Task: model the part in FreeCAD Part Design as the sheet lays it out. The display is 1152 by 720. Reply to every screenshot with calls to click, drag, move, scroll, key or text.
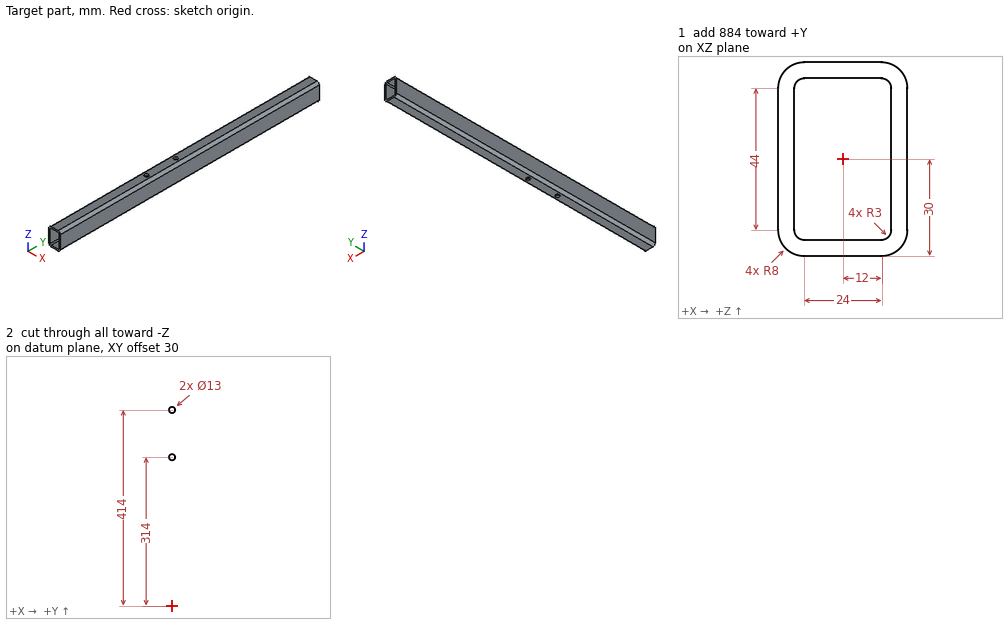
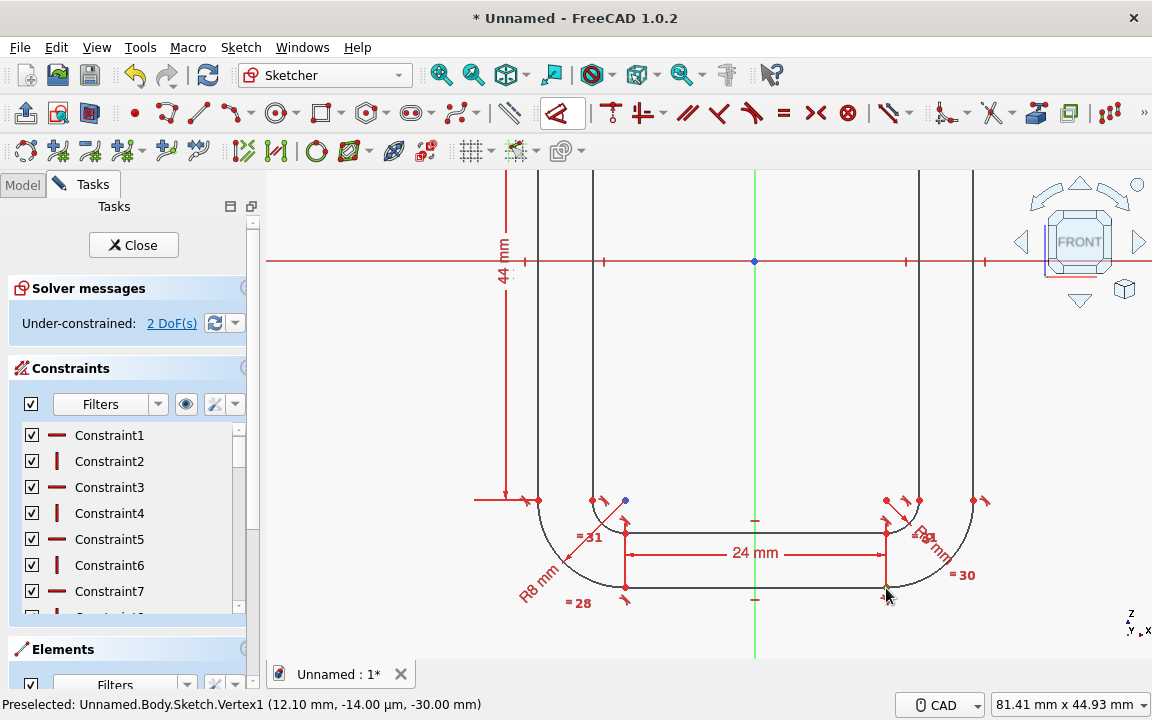
key(l)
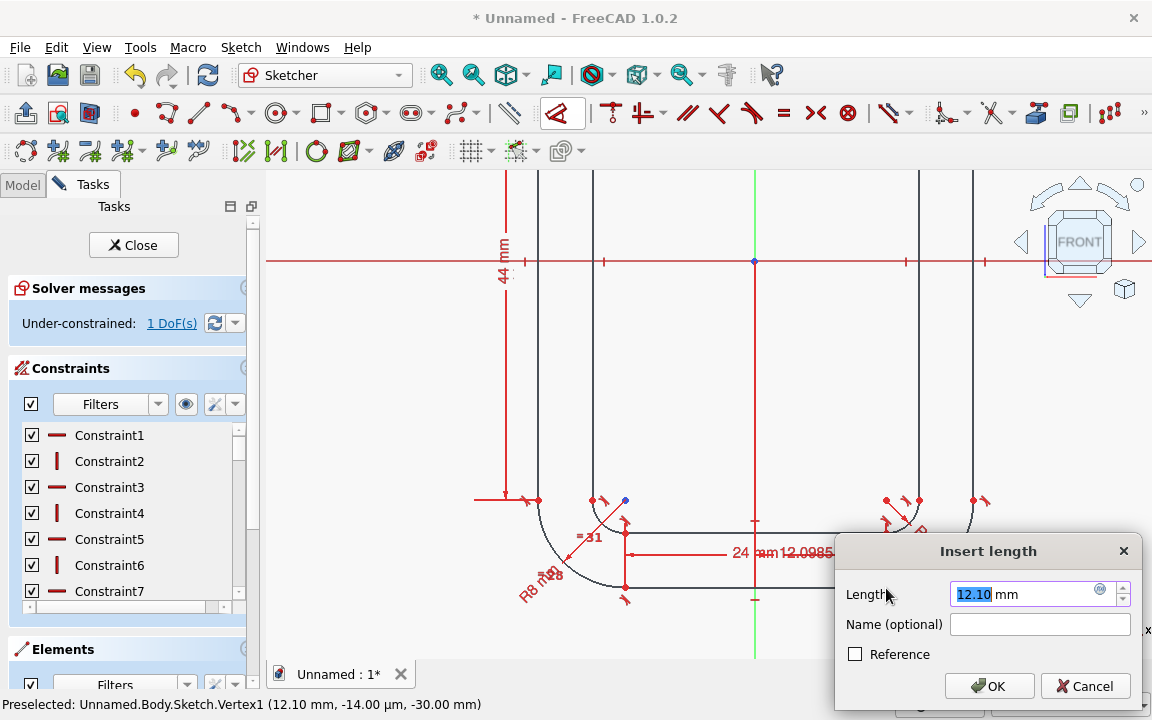
text(12)
key(Return)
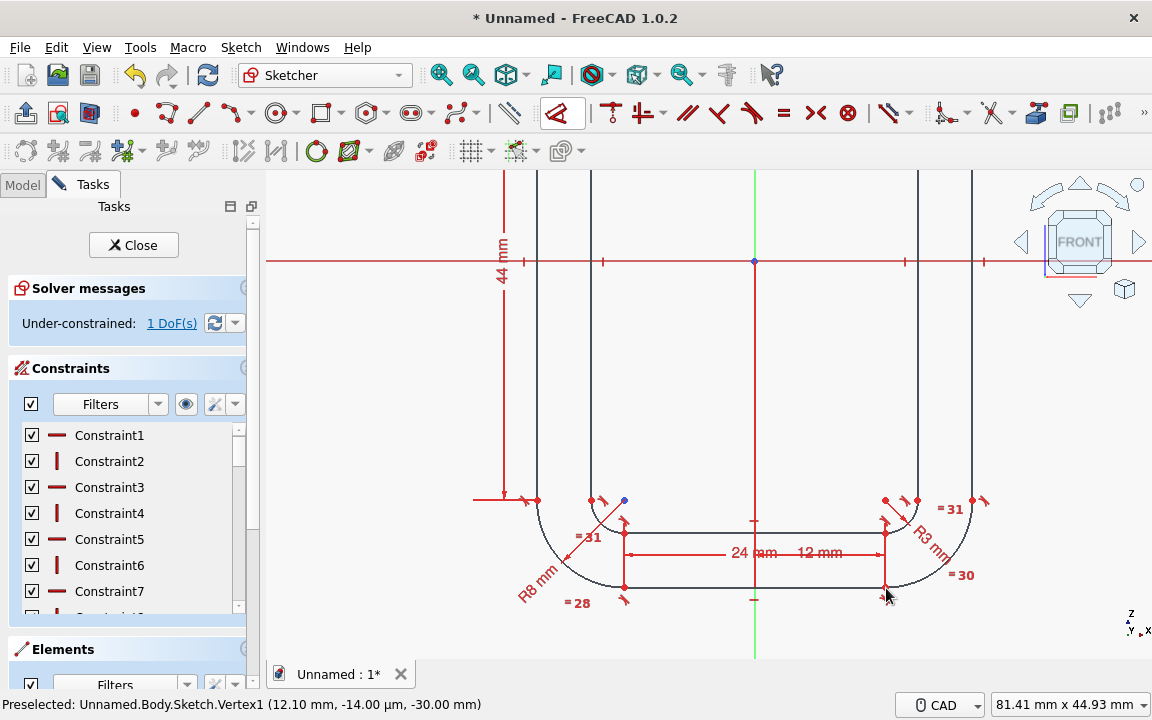
click(885, 588)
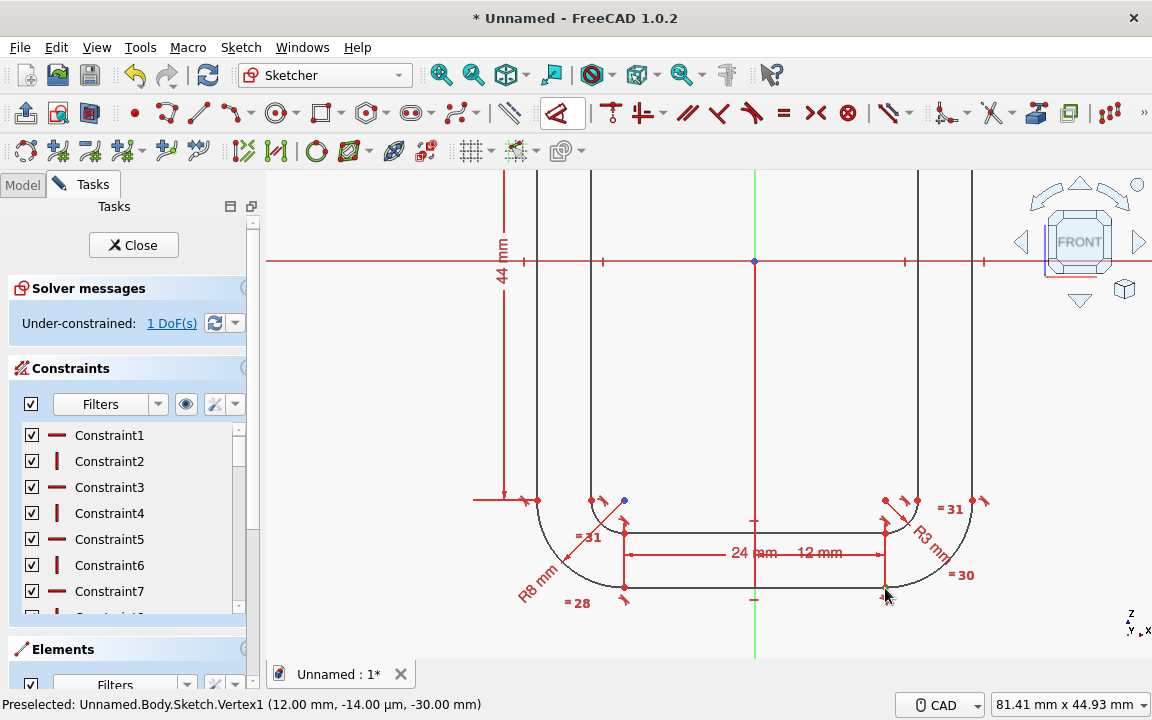
key(i)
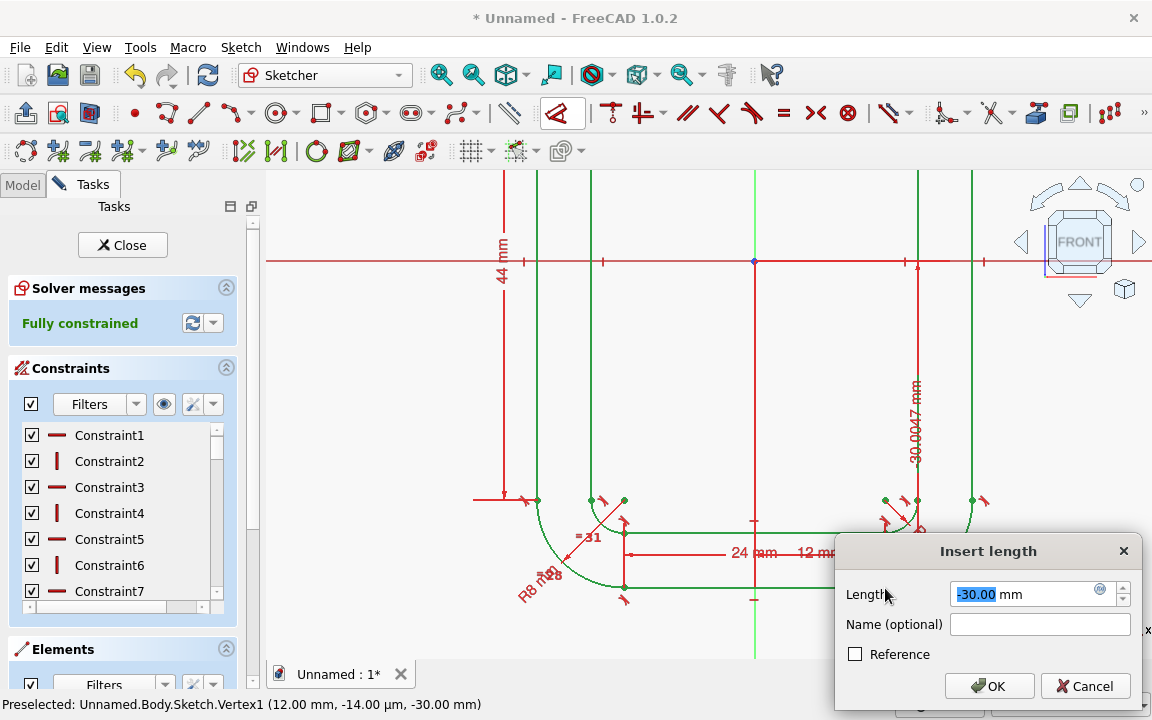
text(-30)
key(Return)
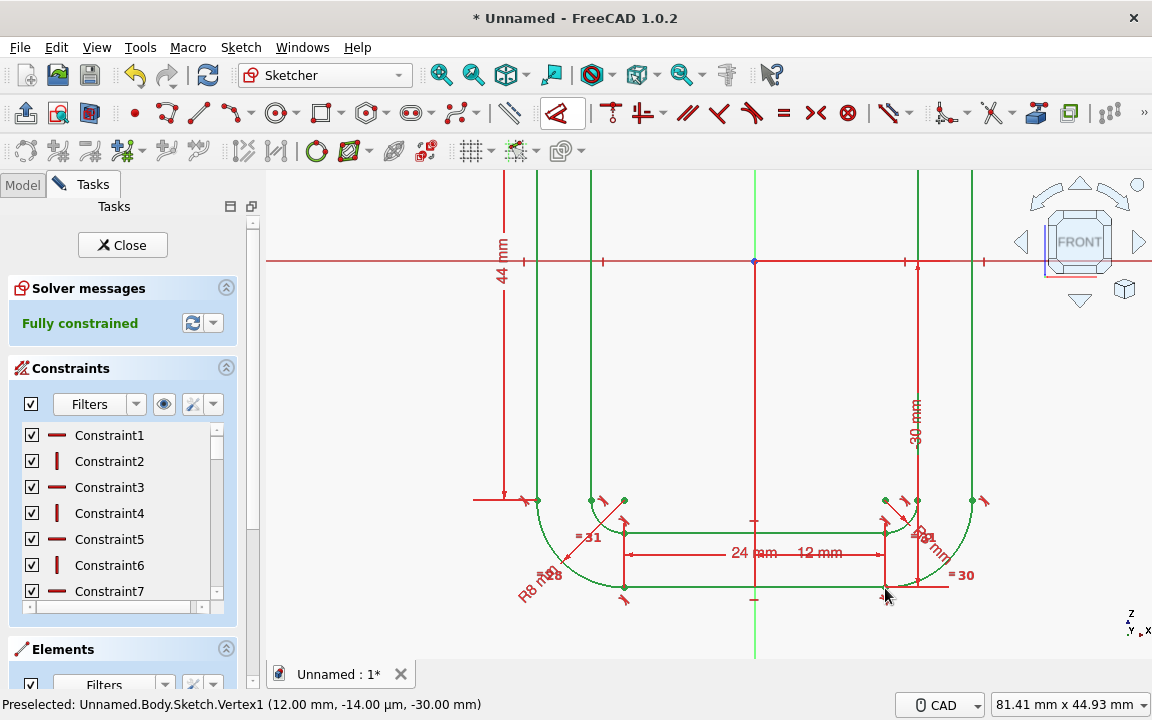
click(123, 245)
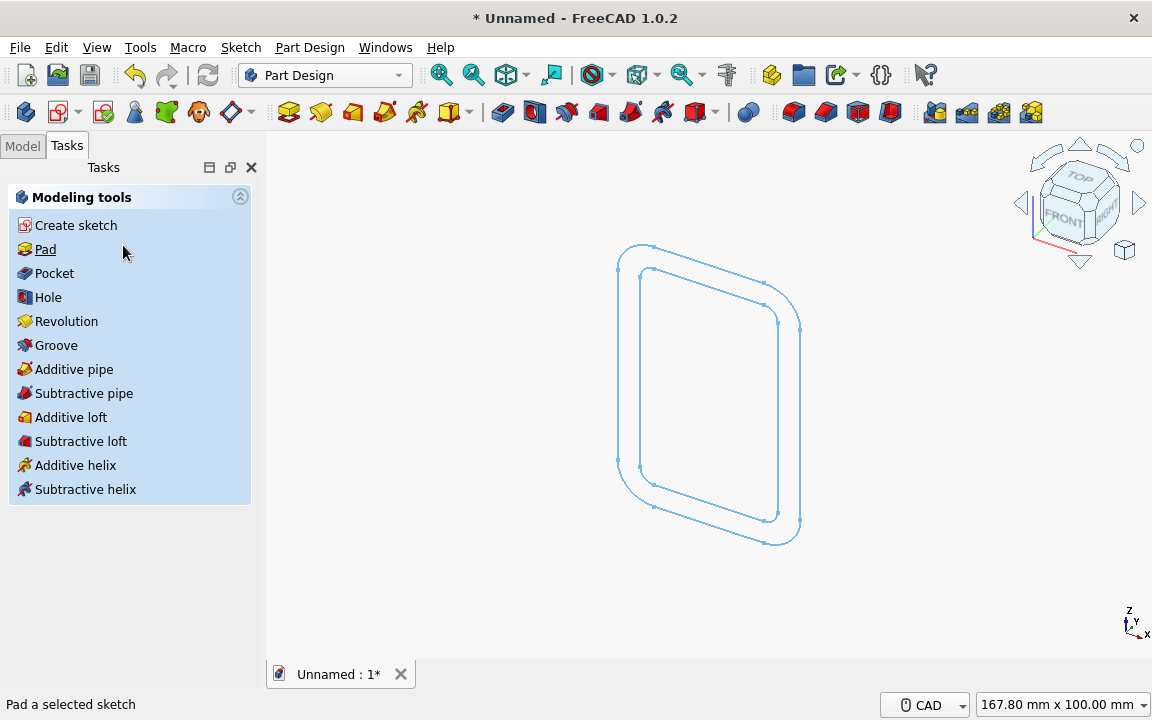
click(290, 112)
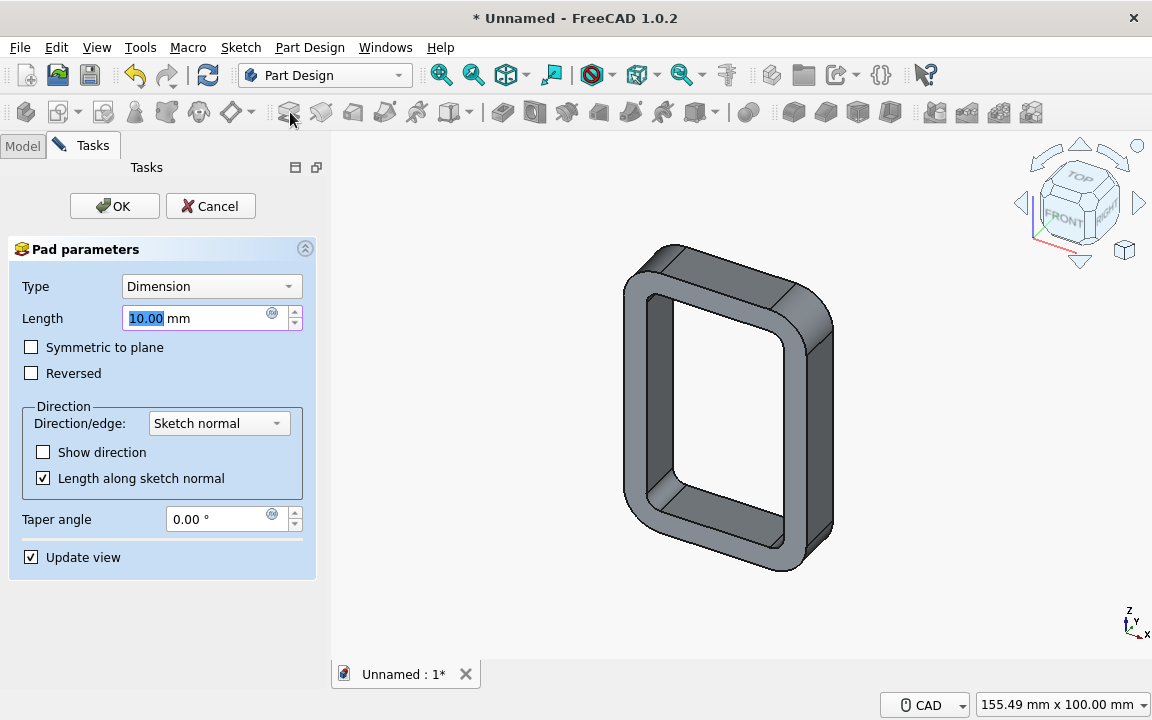
text(884)
key(Tab)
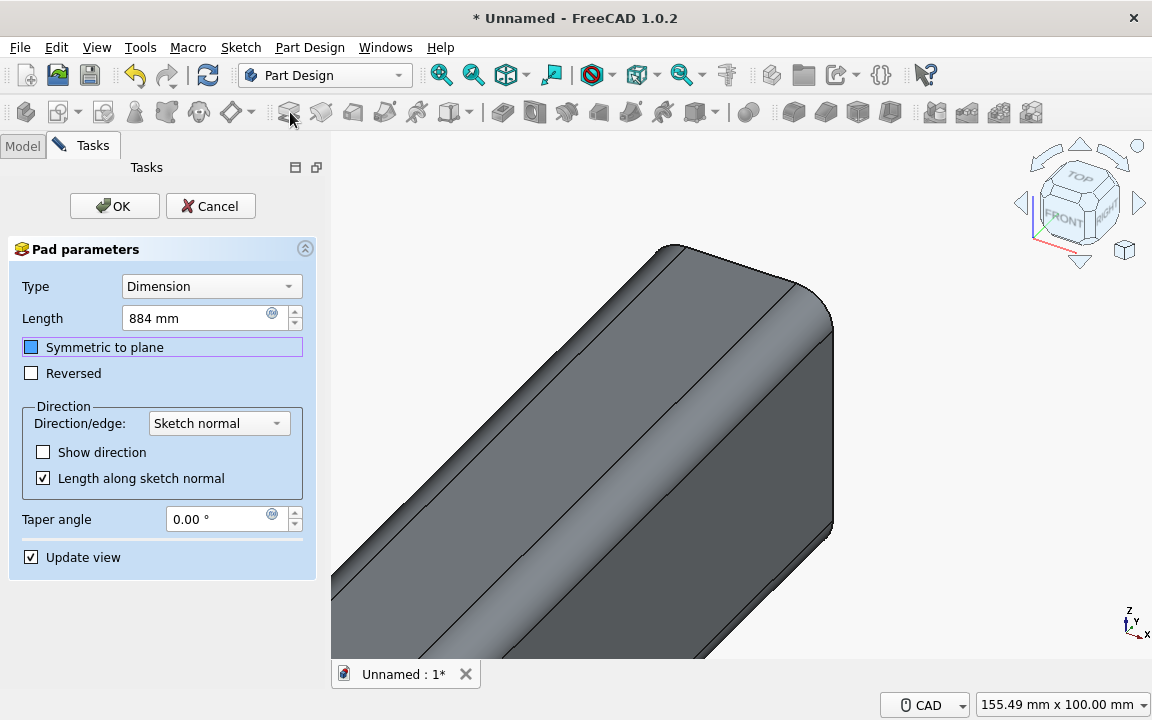
click(30, 373)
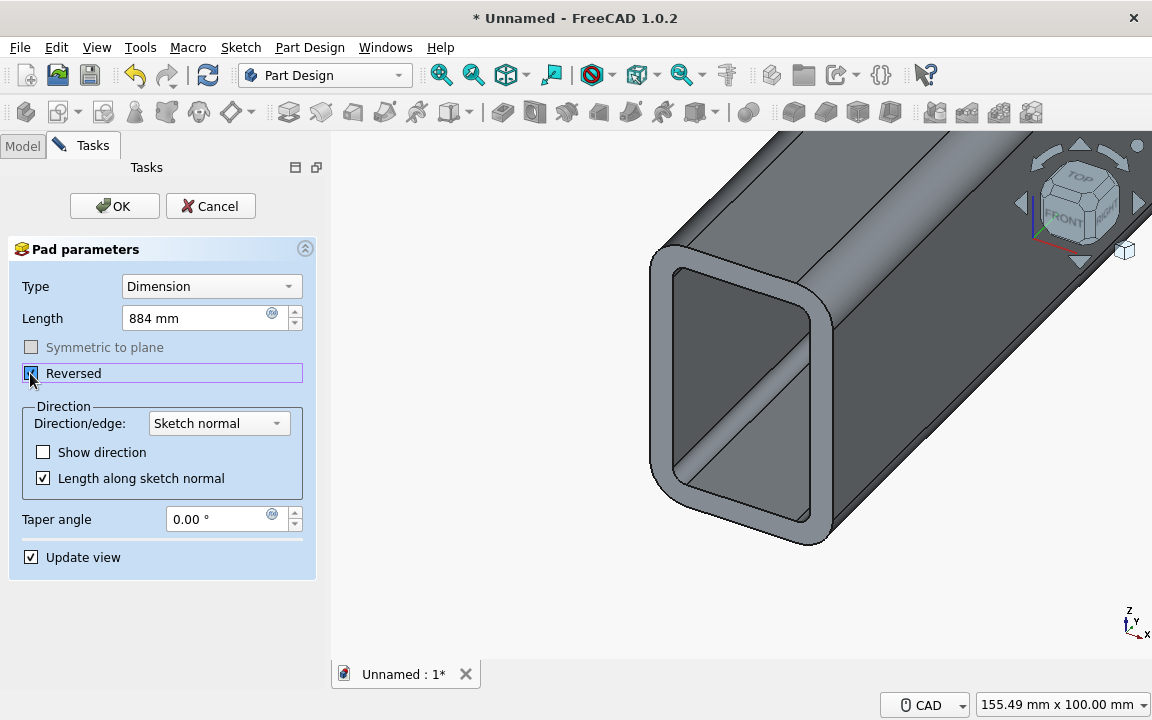
click(115, 206)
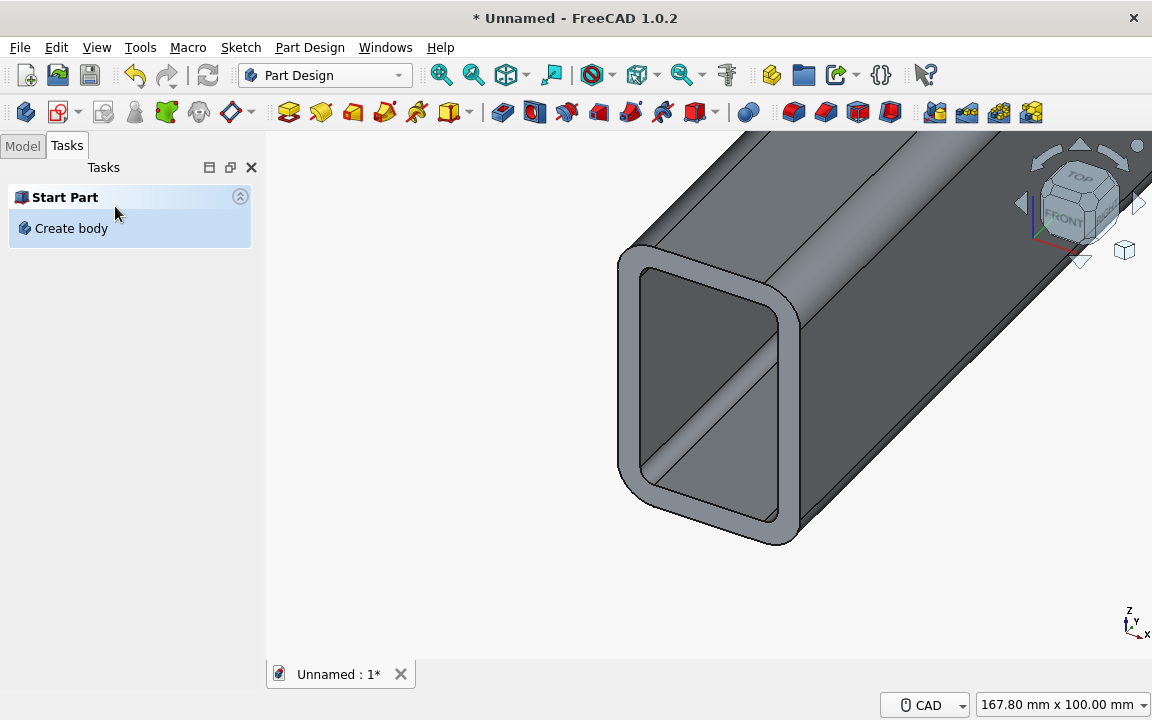
click(442, 76)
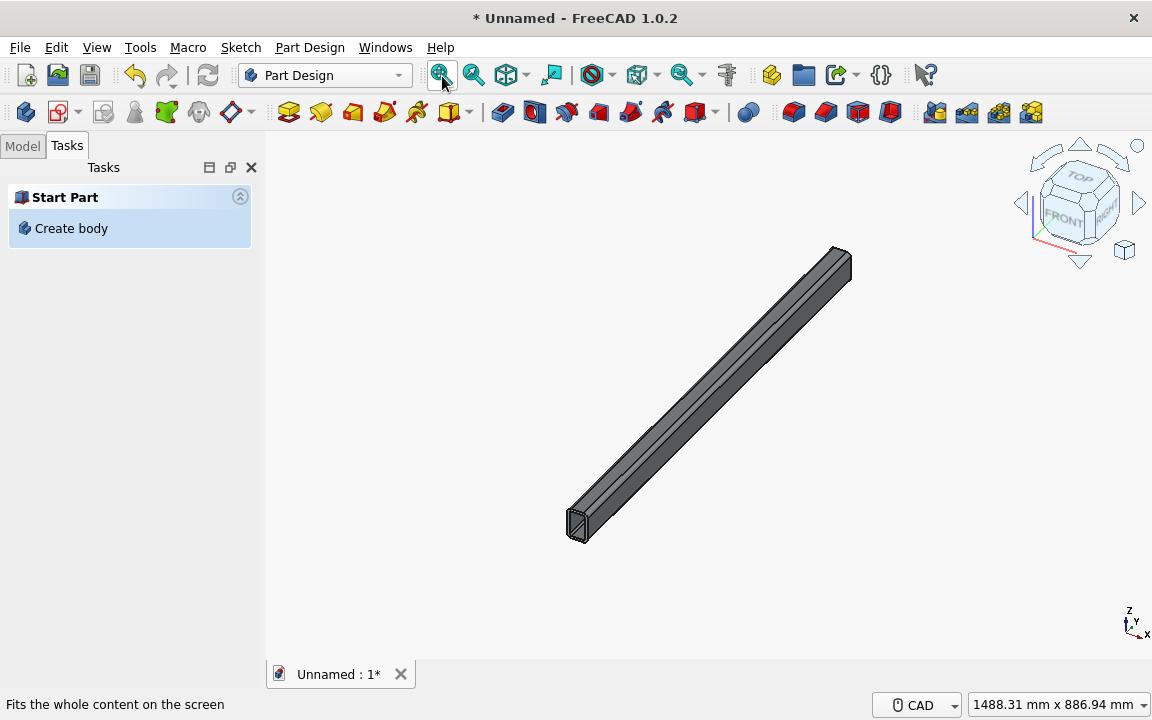
key(0)